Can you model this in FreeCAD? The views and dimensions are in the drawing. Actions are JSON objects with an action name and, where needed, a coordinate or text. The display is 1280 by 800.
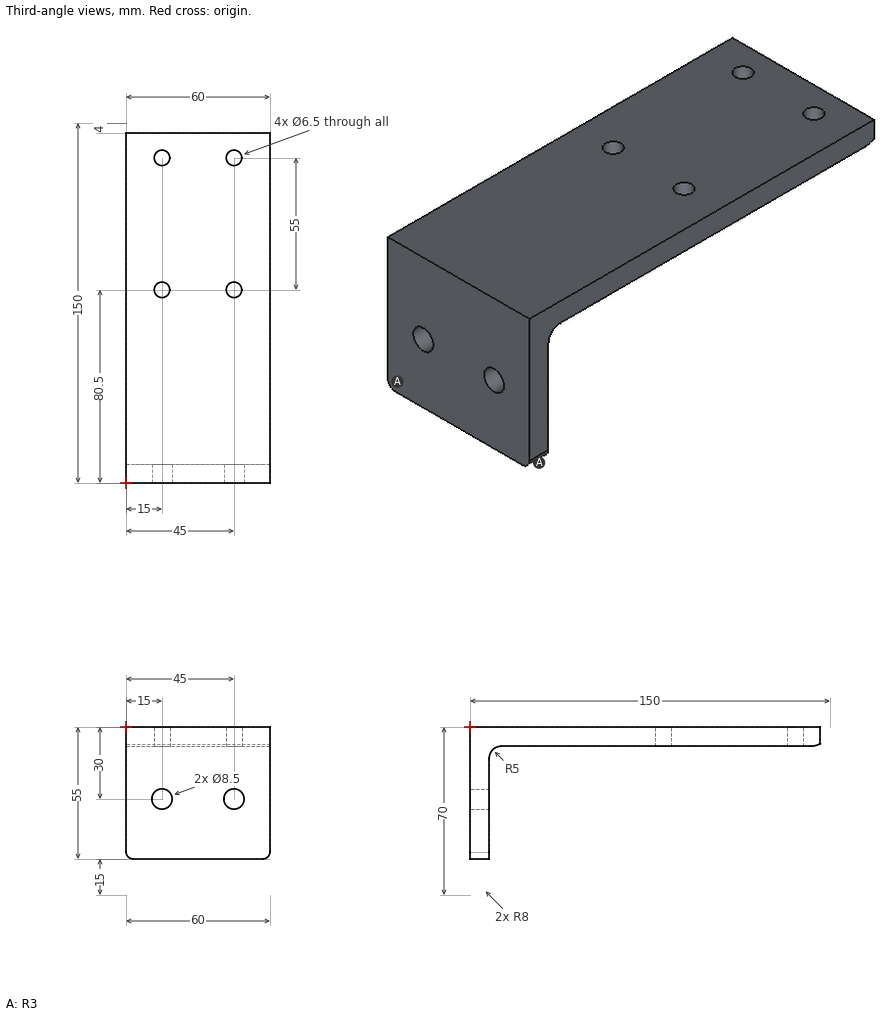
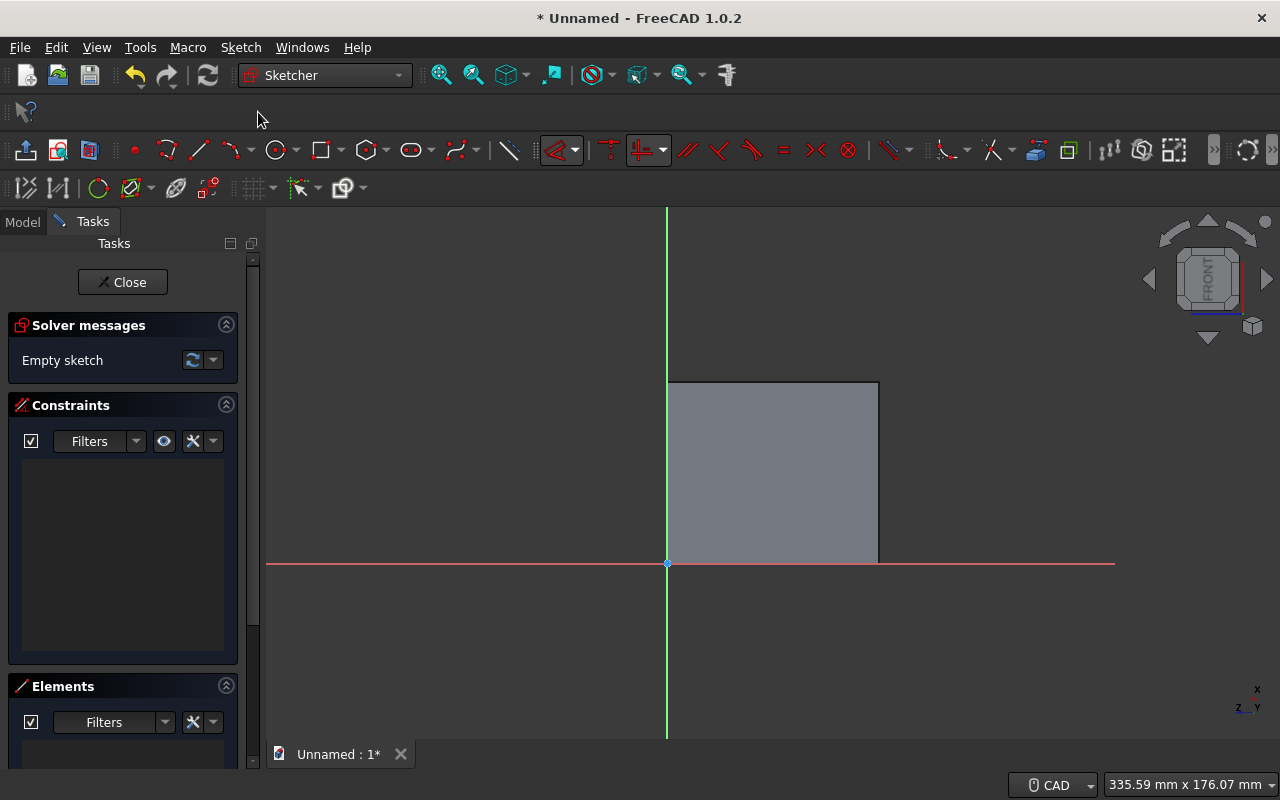
{"action": "scroll", "coordinate": [856, 473], "scroll_direction": "up", "scroll_amount": 3}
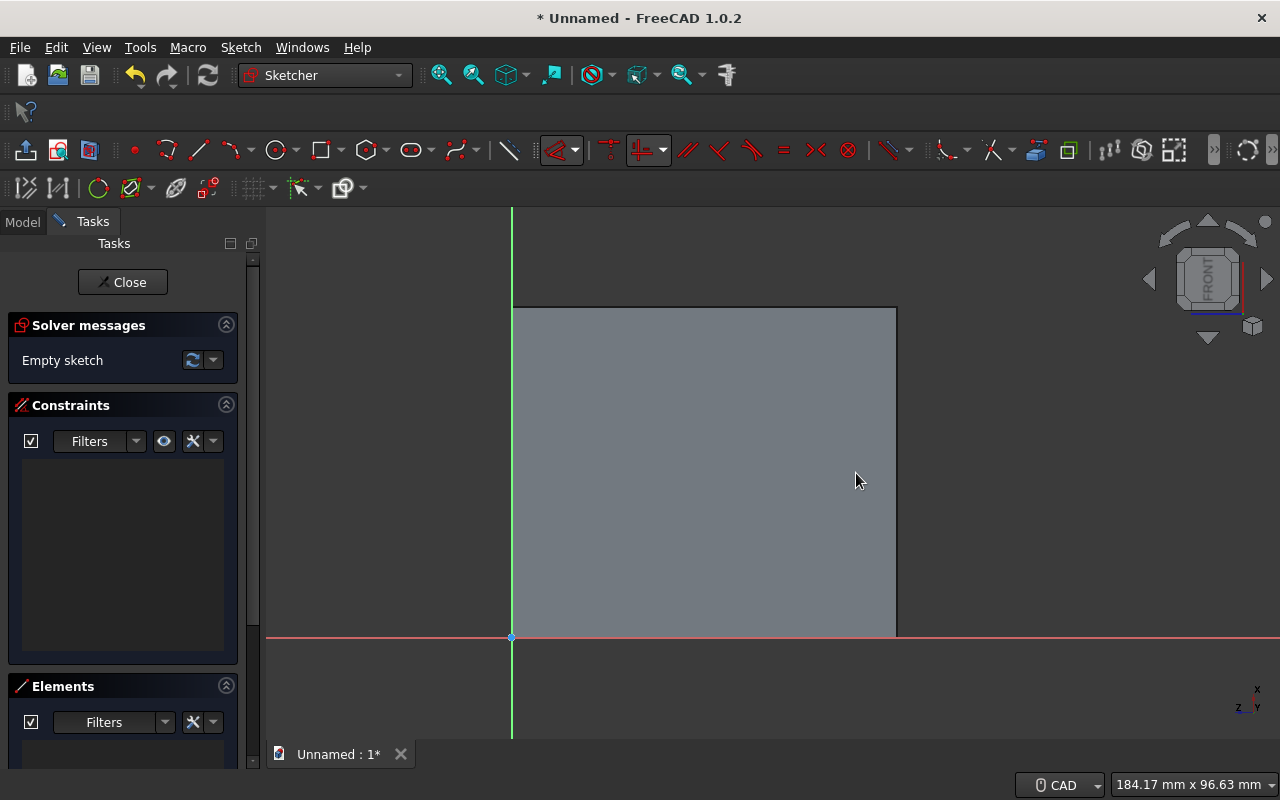
{"action": "key", "text": "g r"}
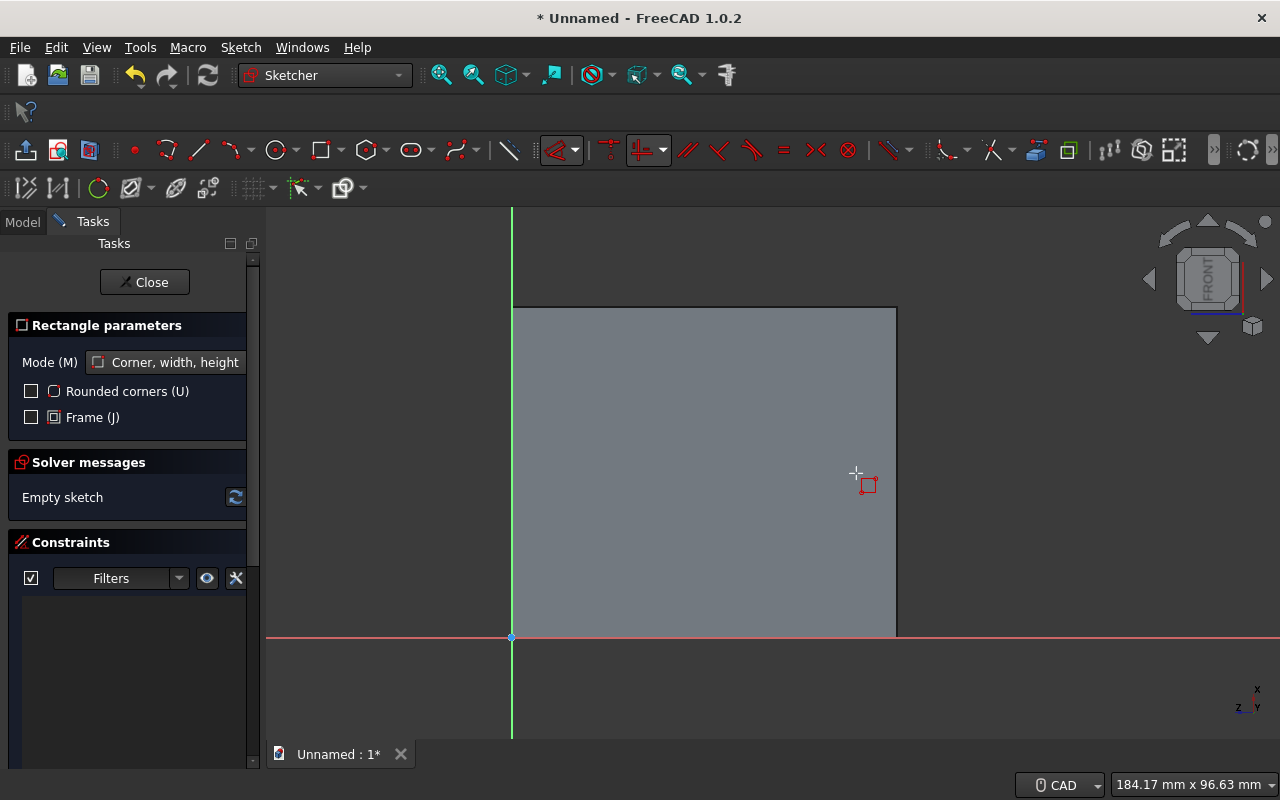
{"action": "left_click", "coordinate": [814, 307]}
{"action": "left_click", "coordinate": [897, 638]}
{"action": "key", "text": "Escape"}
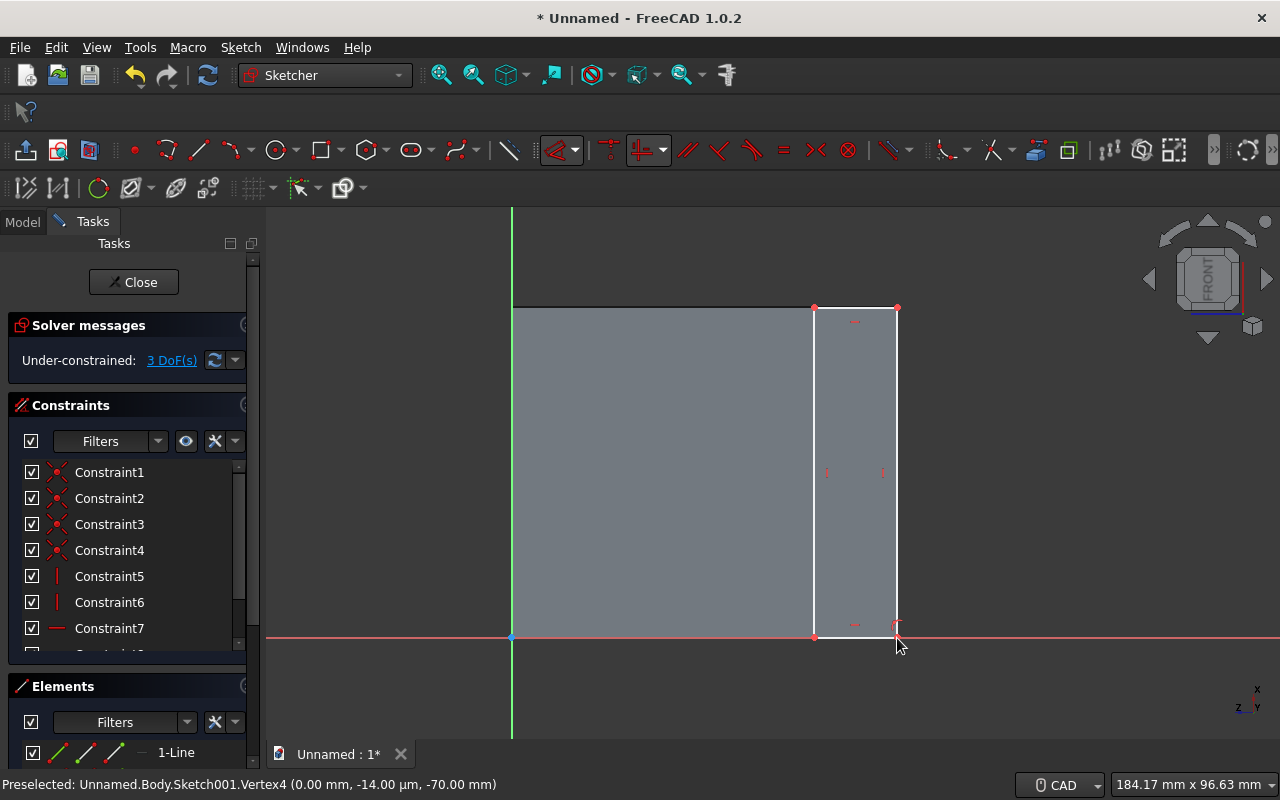
{"action": "left_click", "coordinate": [556, 150]}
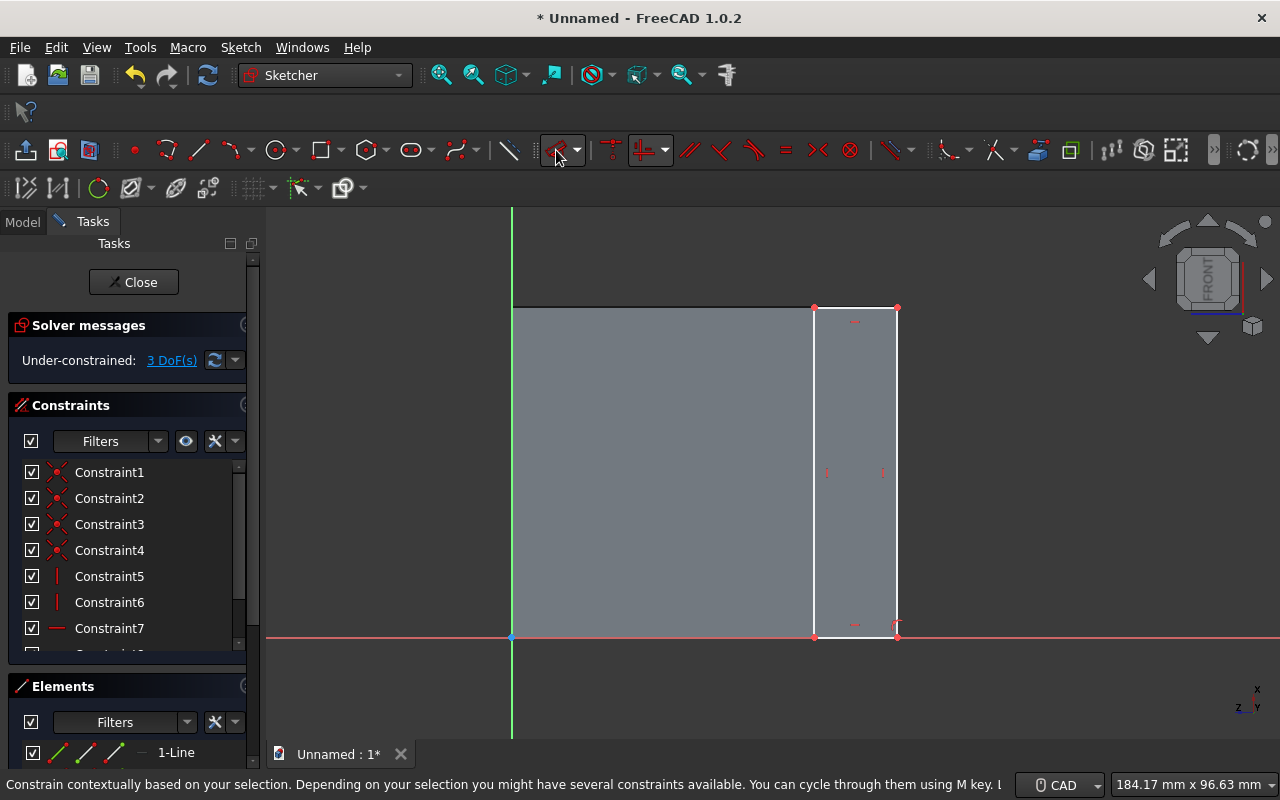
{"action": "left_click", "coordinate": [814, 407]}
{"action": "left_click", "coordinate": [848, 473]}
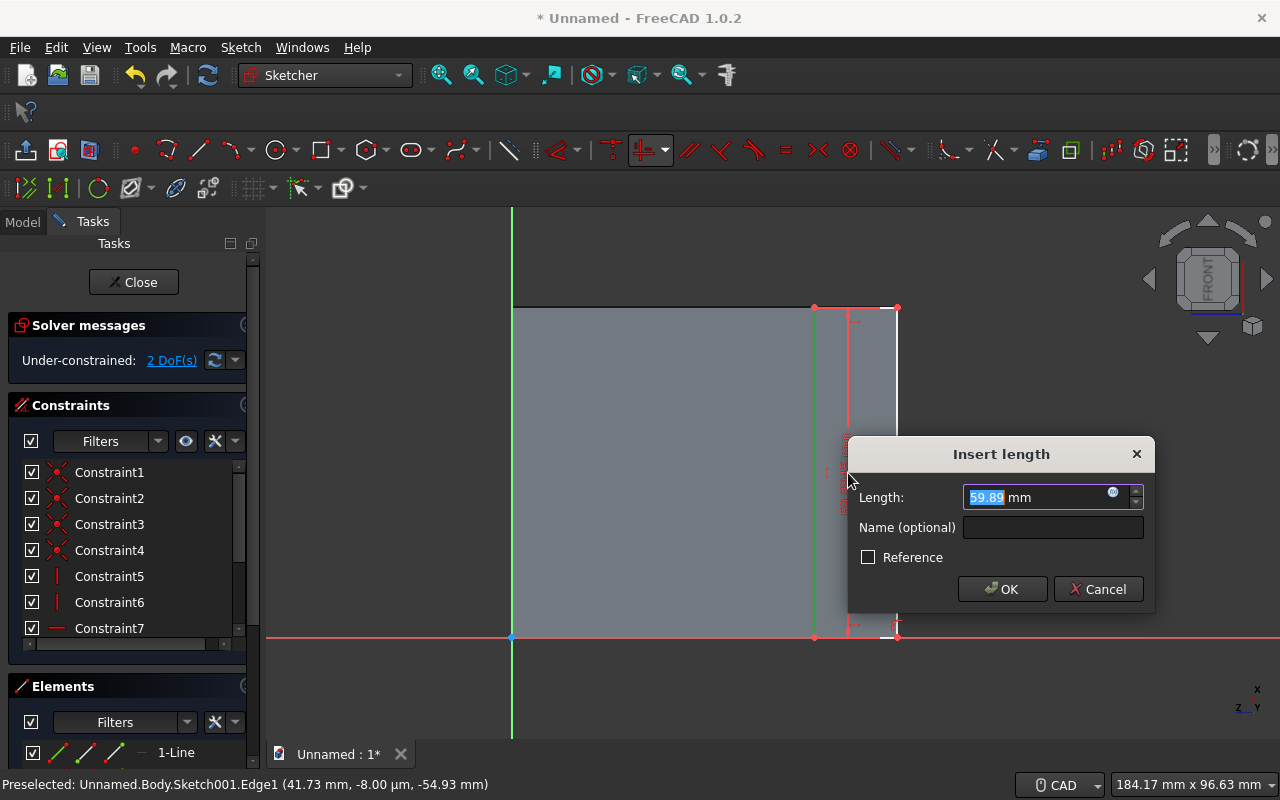
{"action": "type", "text": "60"}
{"action": "key", "text": "Return"}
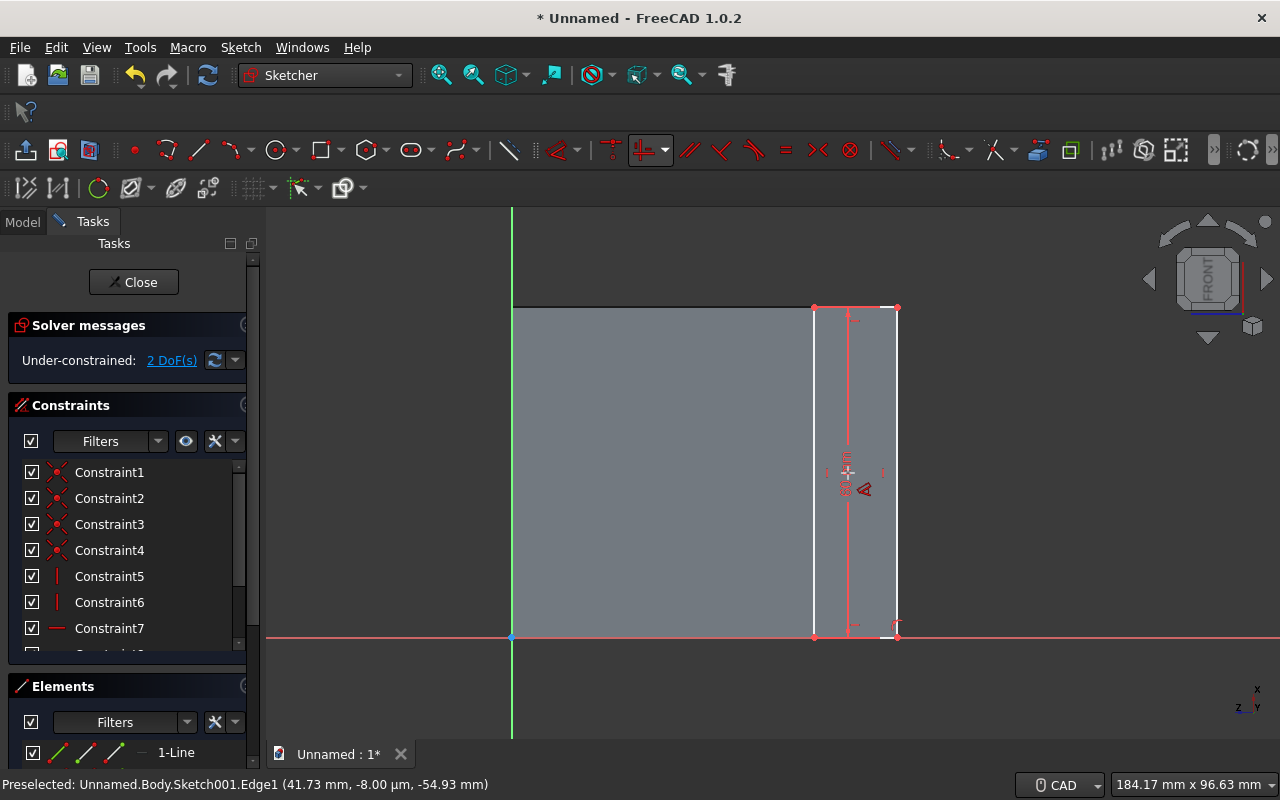
{"action": "left_click", "coordinate": [839, 638]}
{"action": "left_click", "coordinate": [856, 672]}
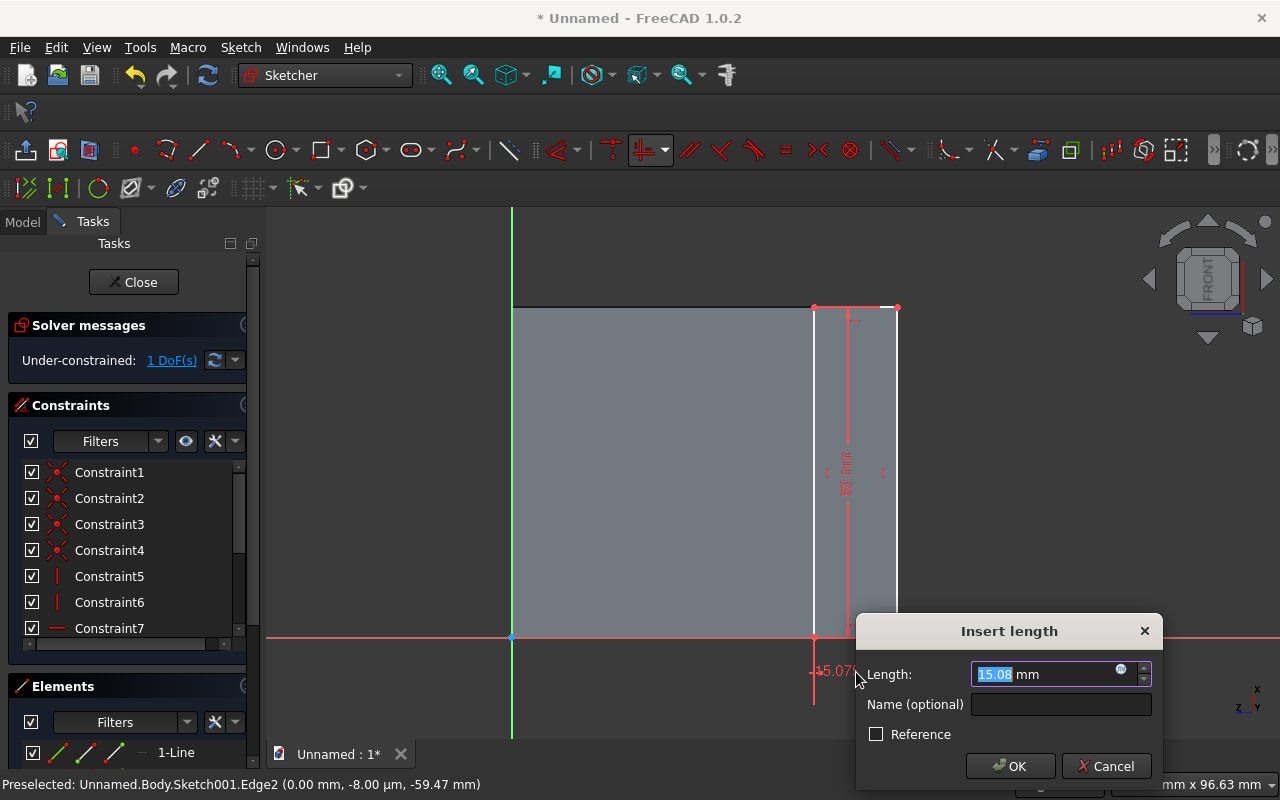
{"action": "type", "text": "15"}
{"action": "key", "text": "Return"}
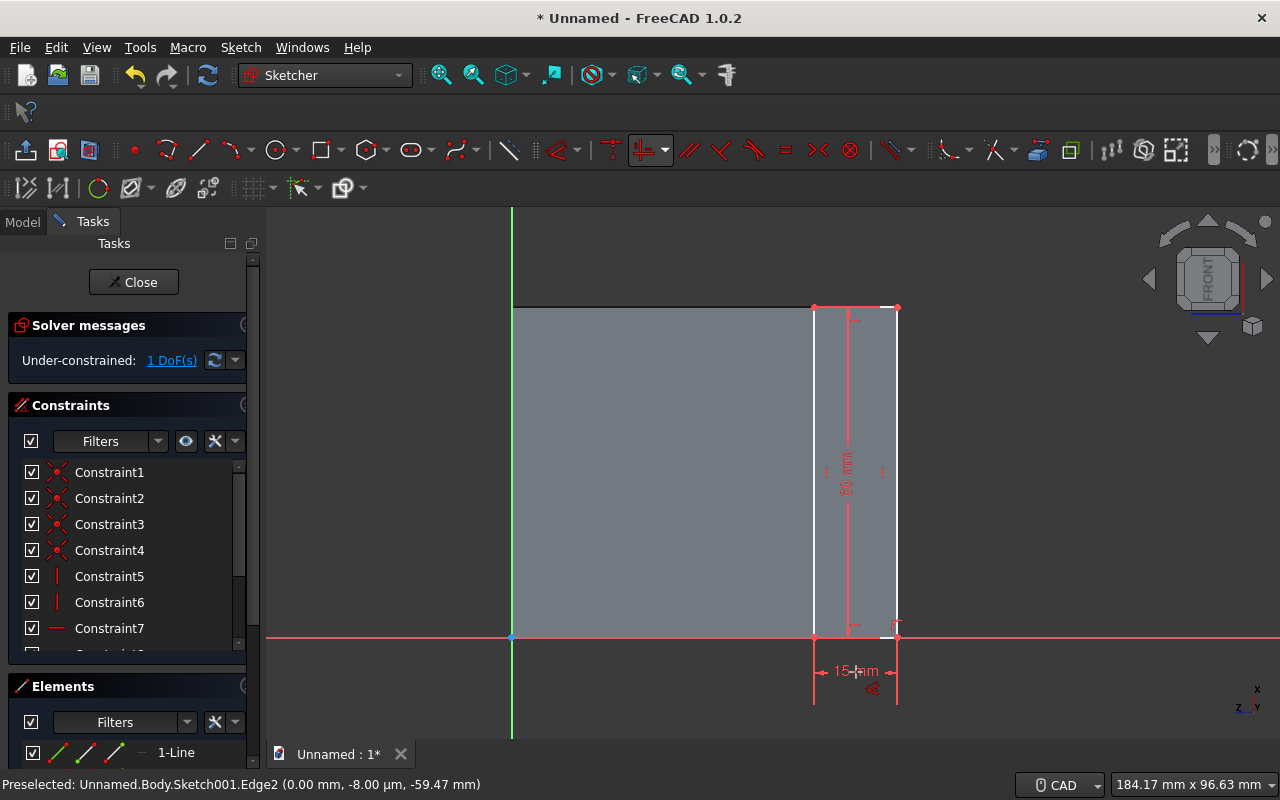
{"action": "left_click", "coordinate": [814, 307]}
{"action": "left_click", "coordinate": [663, 672]}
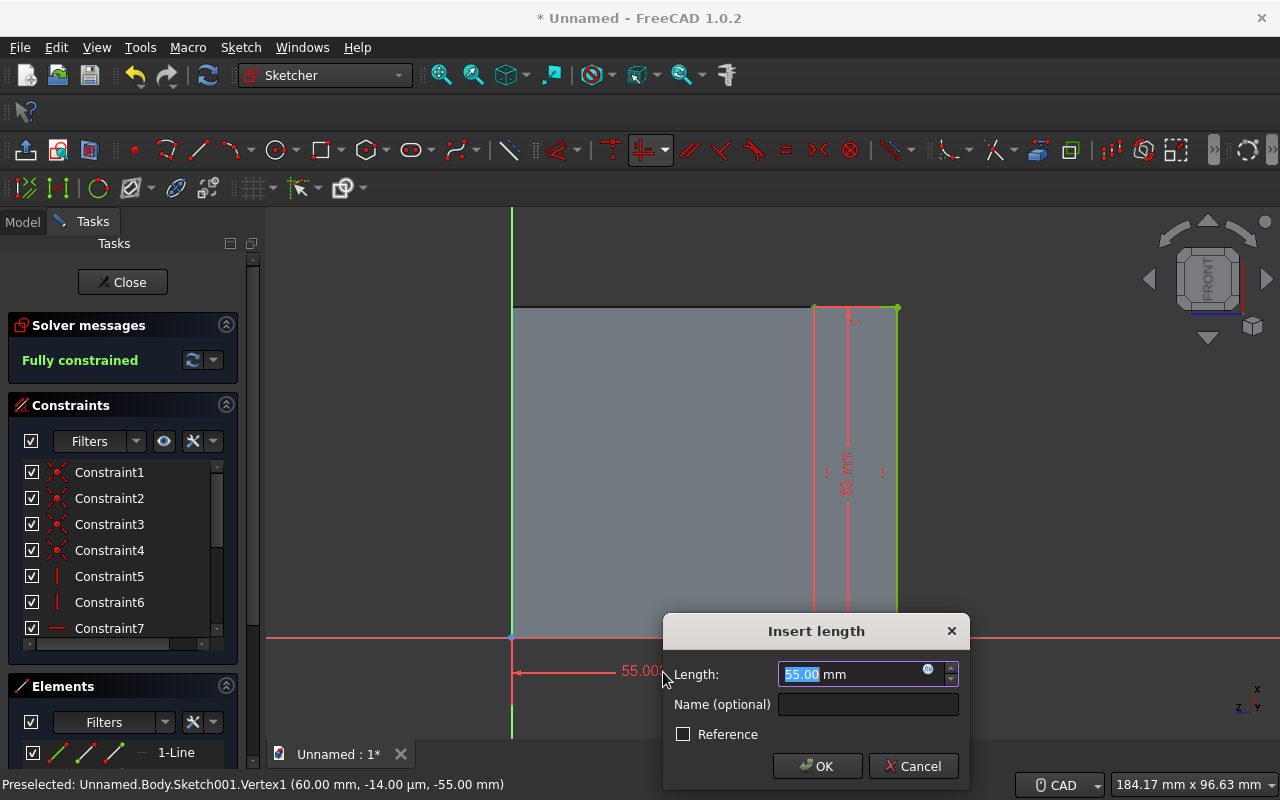
{"action": "type", "text": "55"}
{"action": "key", "text": "Return"}
{"action": "key", "text": "Escape"}